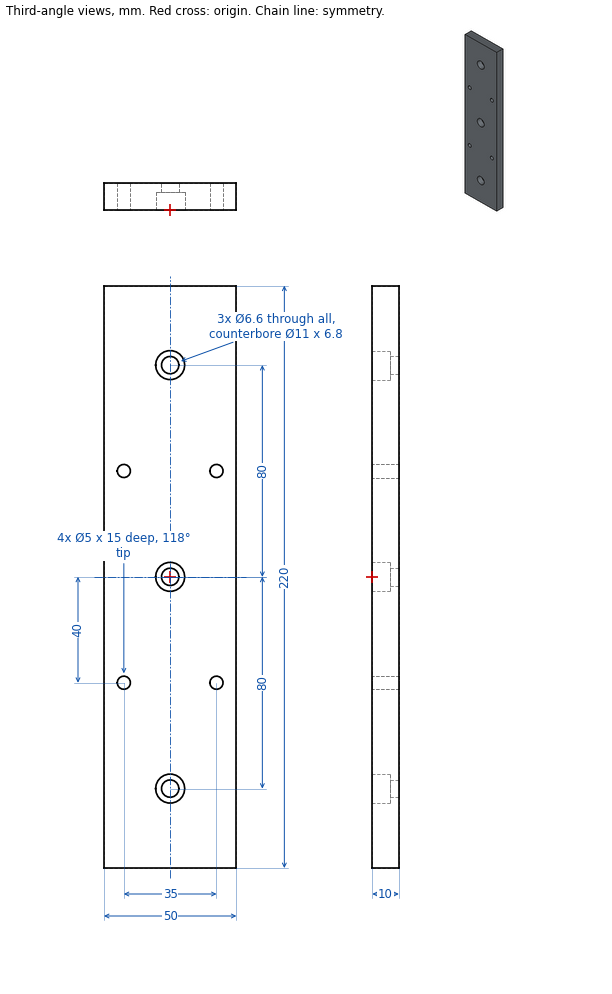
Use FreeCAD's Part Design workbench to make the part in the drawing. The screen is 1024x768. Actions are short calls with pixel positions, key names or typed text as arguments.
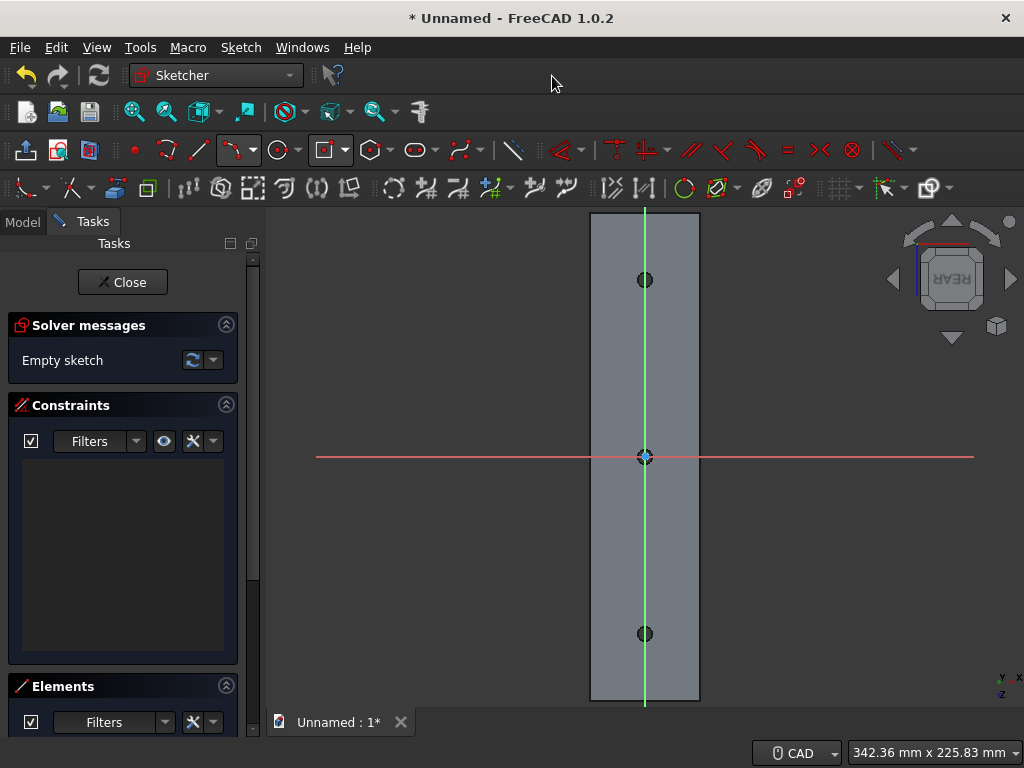
scroll(728, 457, up, 3)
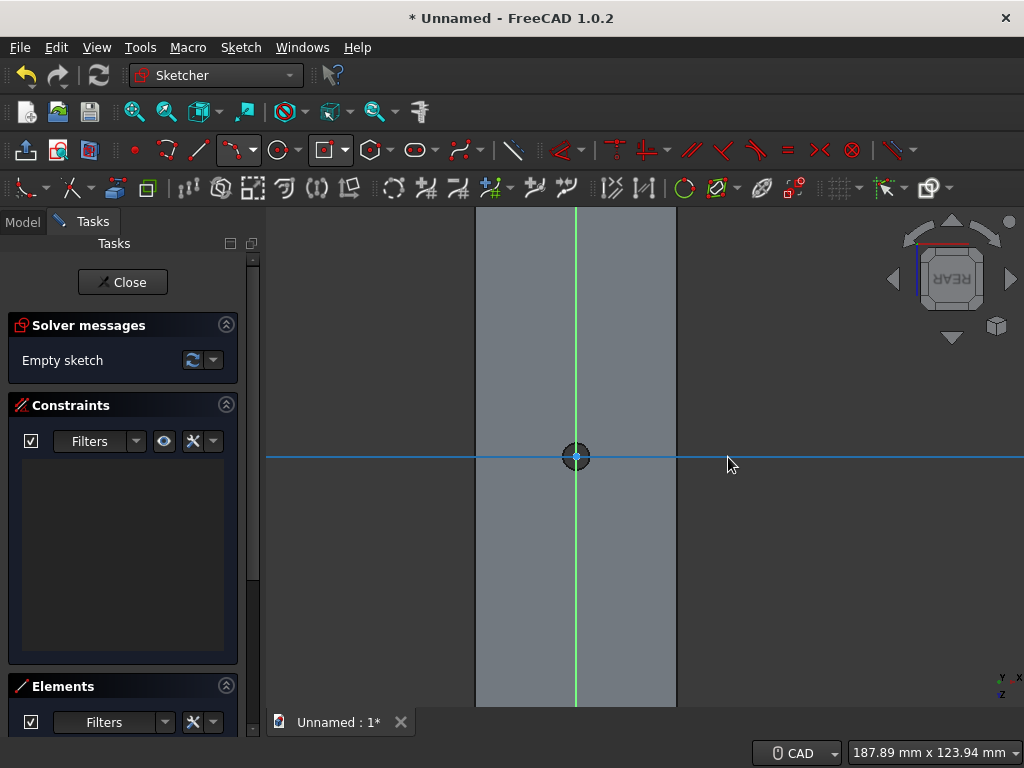
click(278, 150)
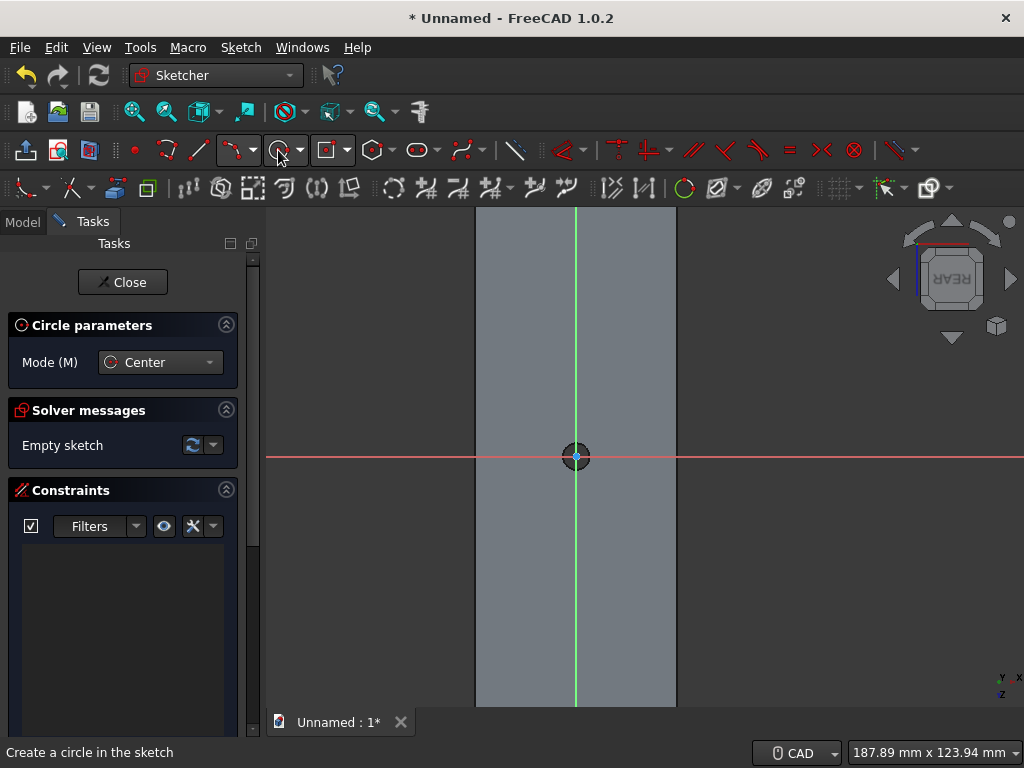
scroll(506, 295, up, 5)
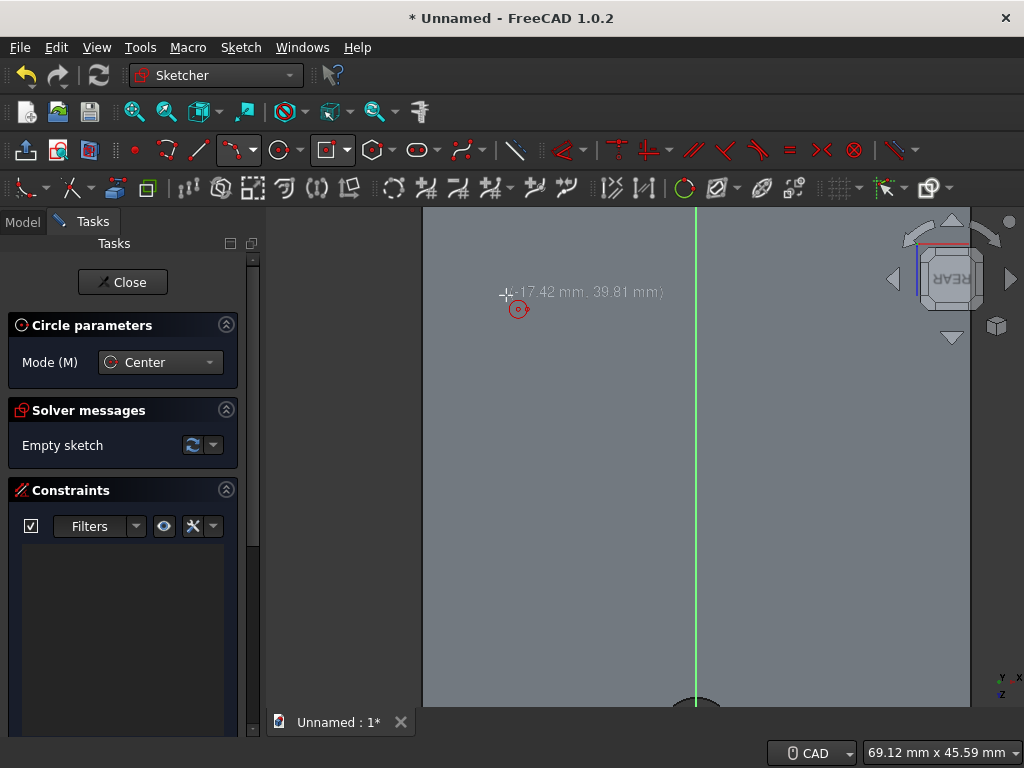
click(505, 295)
move(524, 276)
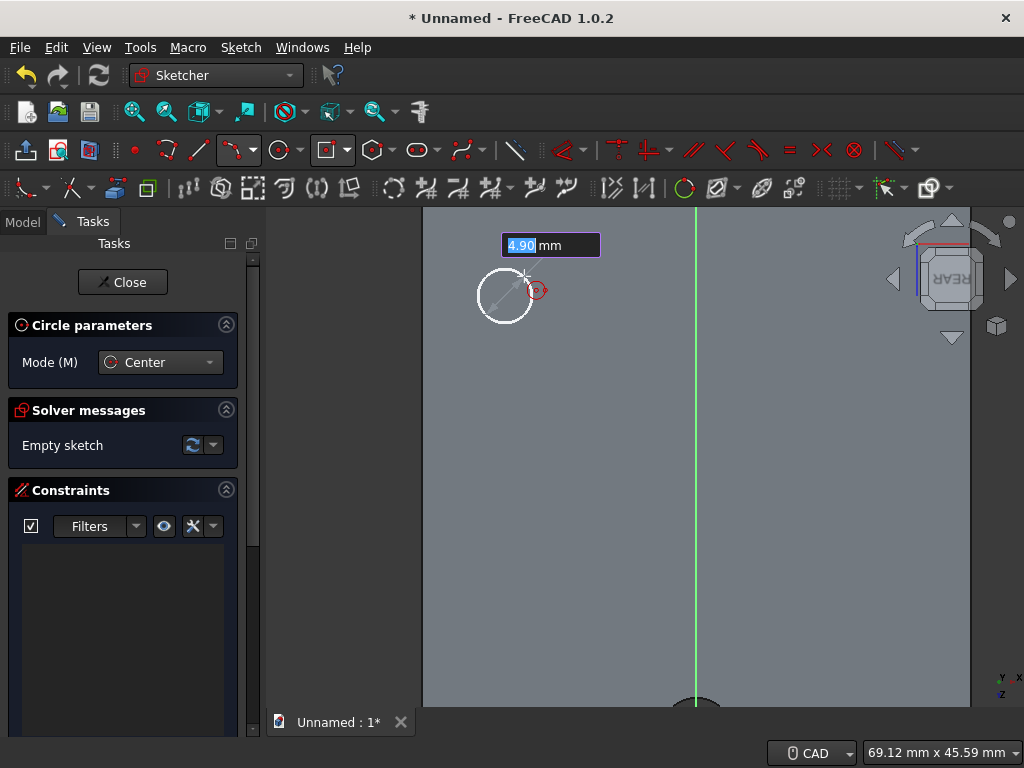
text(5)
key(Return)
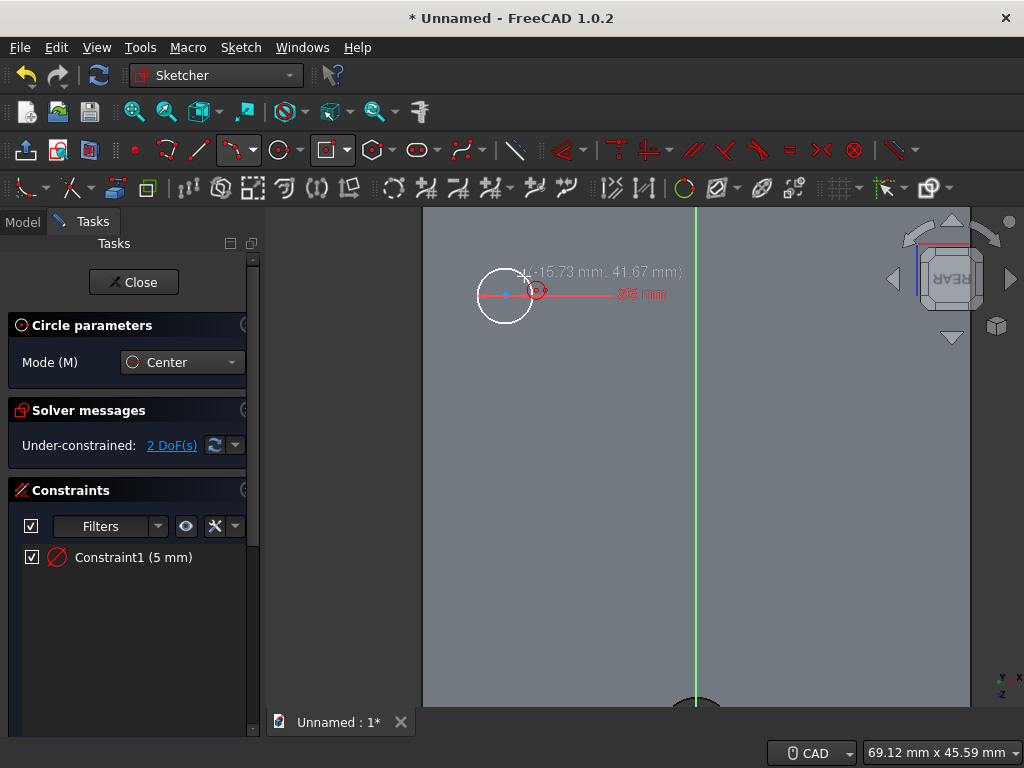
scroll(507, 296, down, 5)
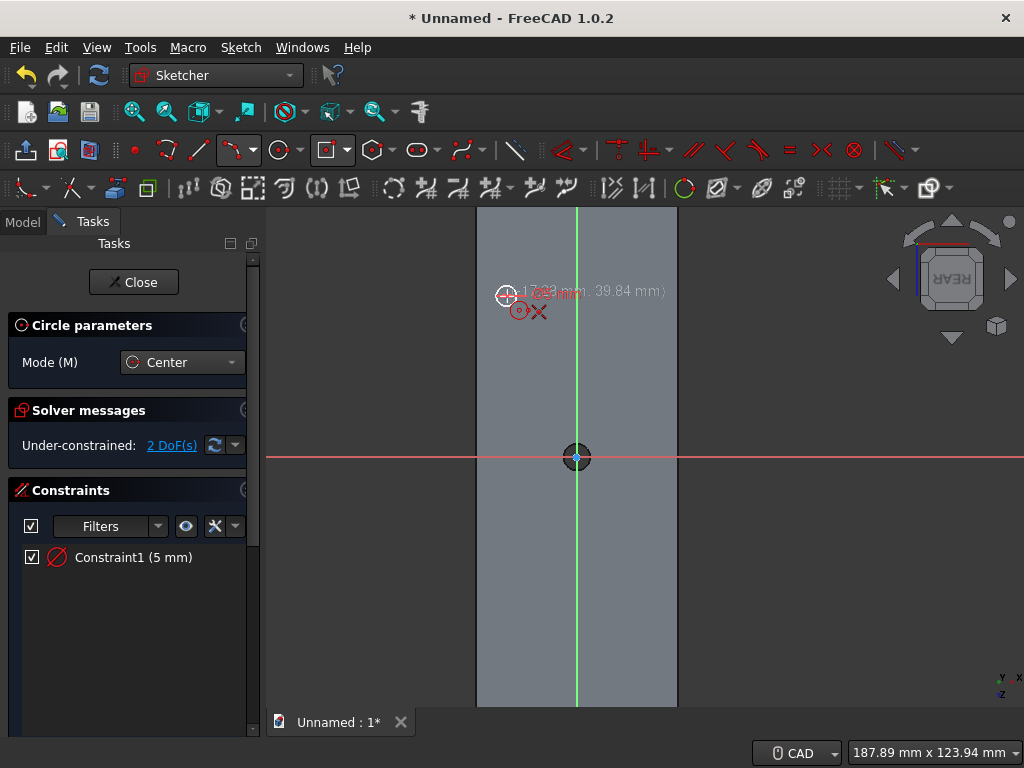
scroll(506, 619, up, 5)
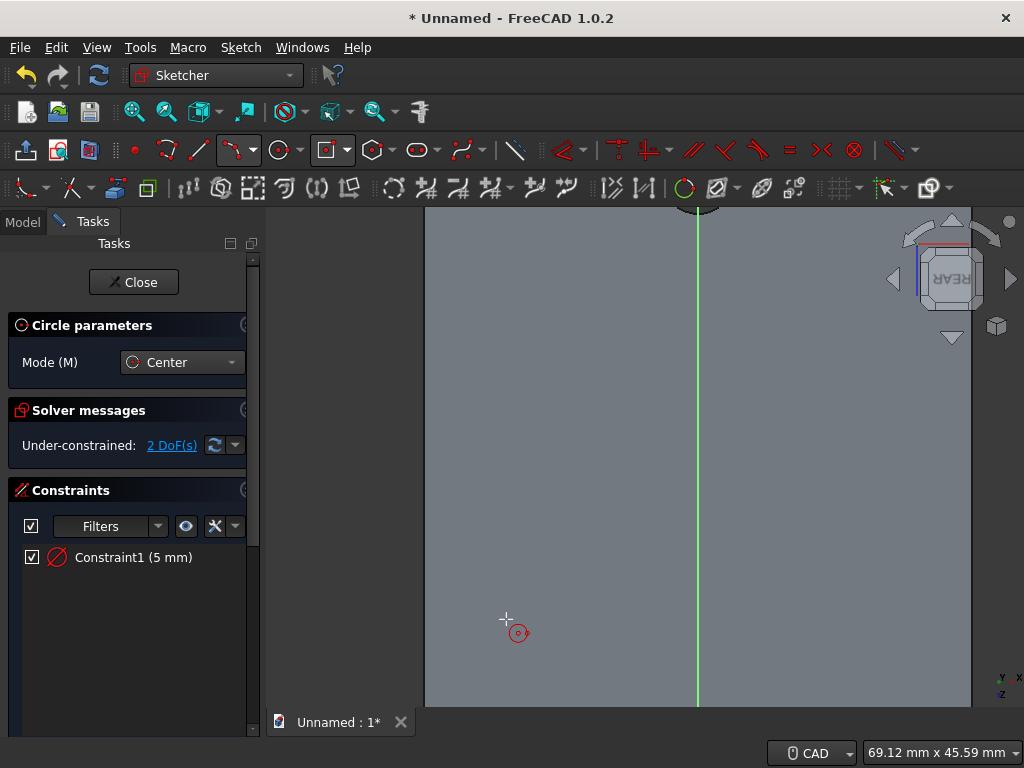
click(506, 616)
move(526, 597)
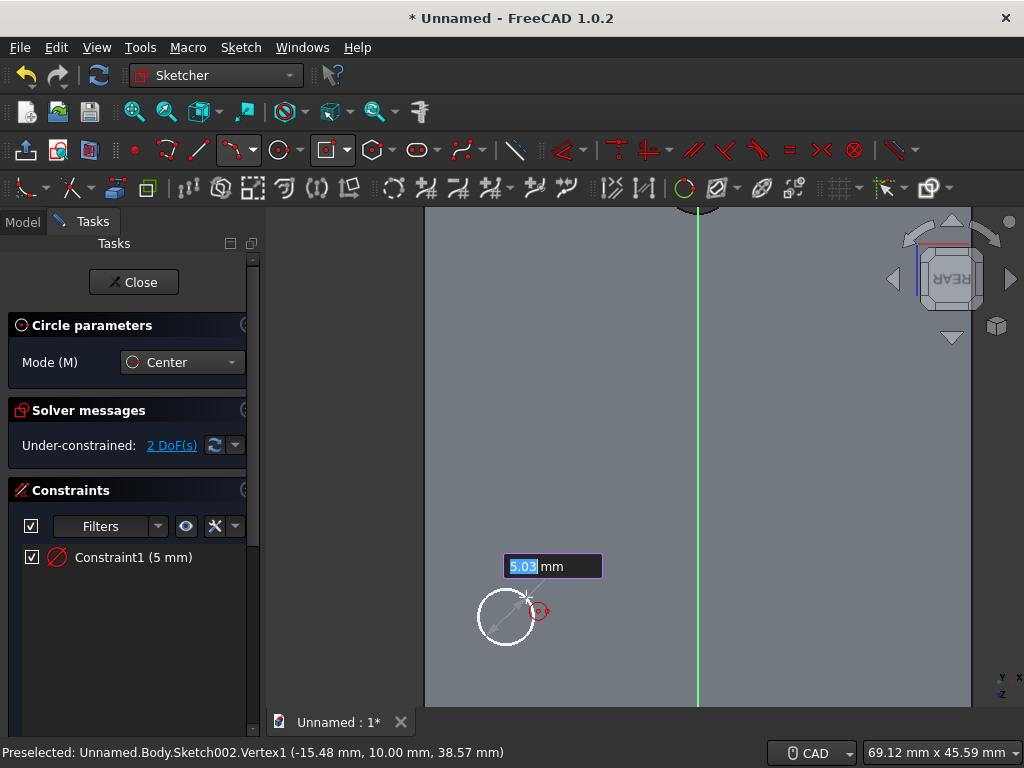
text(5)
key(Return)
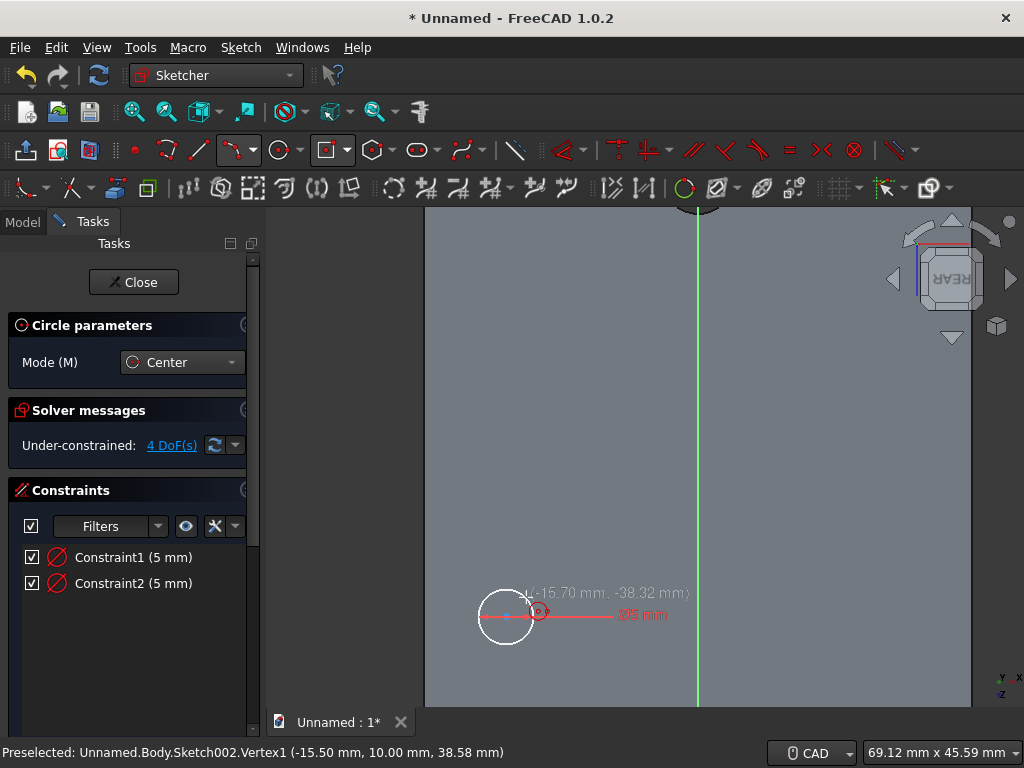
scroll(506, 619, down, 5)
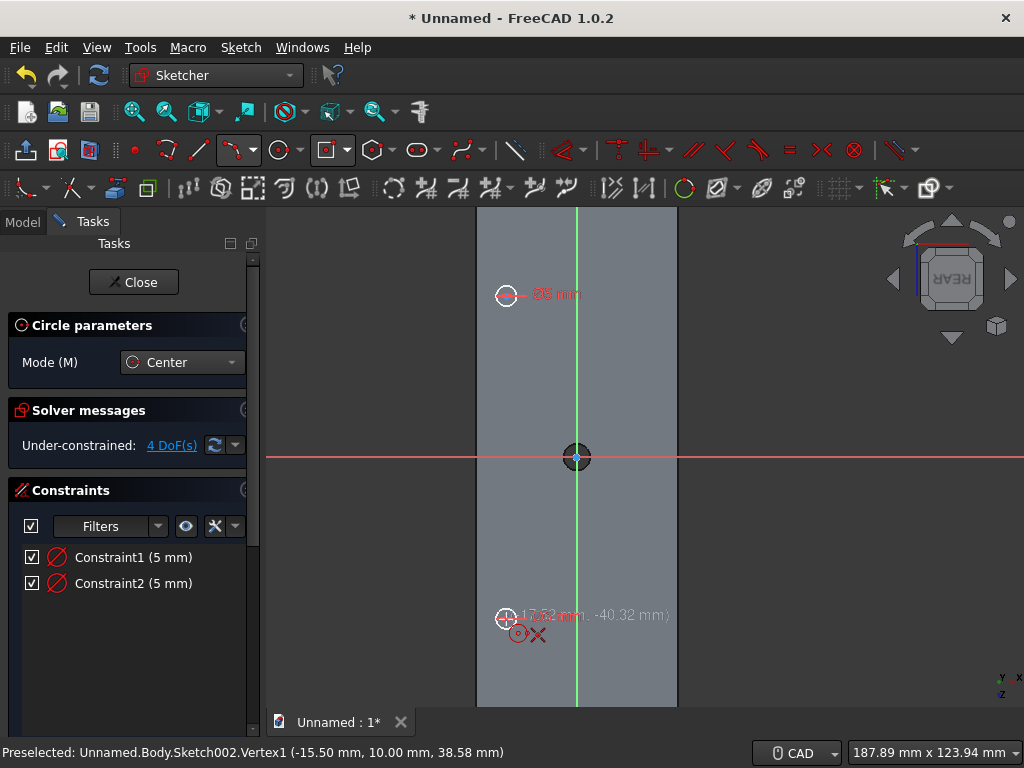
scroll(647, 296, up, 5)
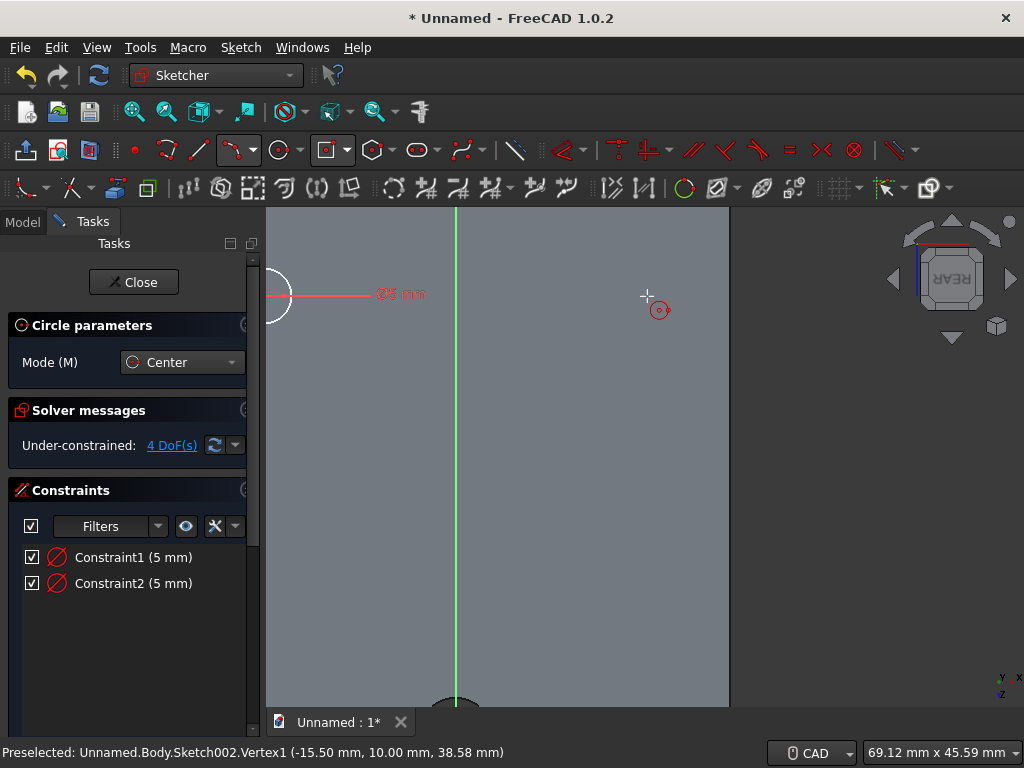
click(647, 295)
move(667, 276)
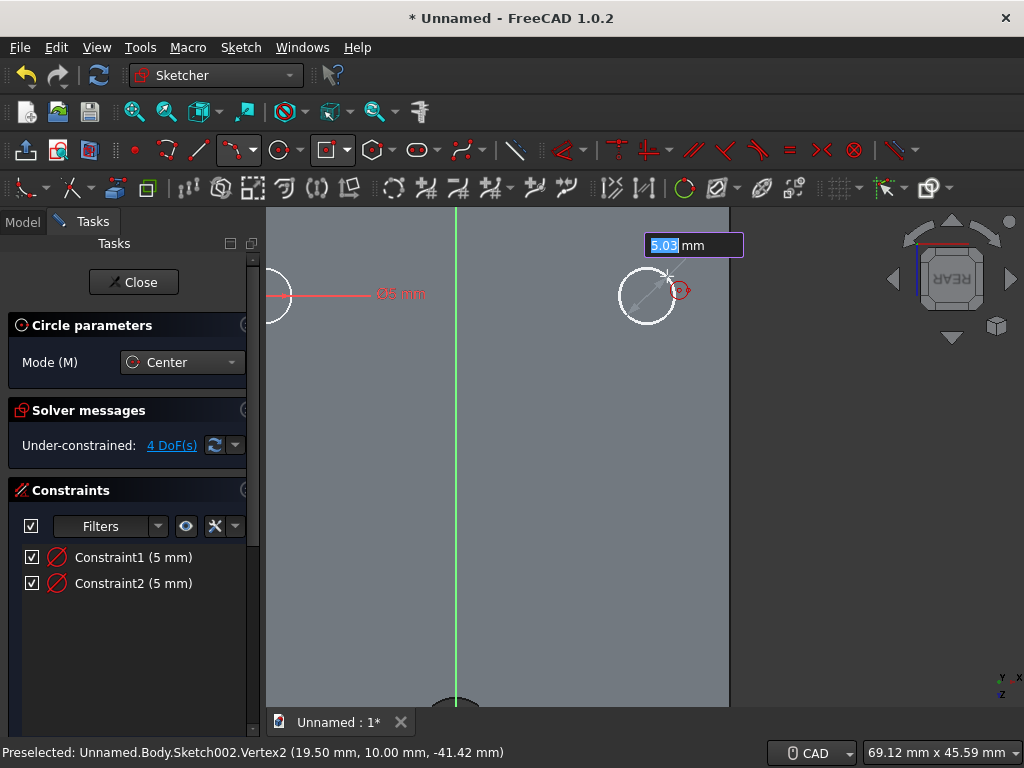
text(5)
key(Return)